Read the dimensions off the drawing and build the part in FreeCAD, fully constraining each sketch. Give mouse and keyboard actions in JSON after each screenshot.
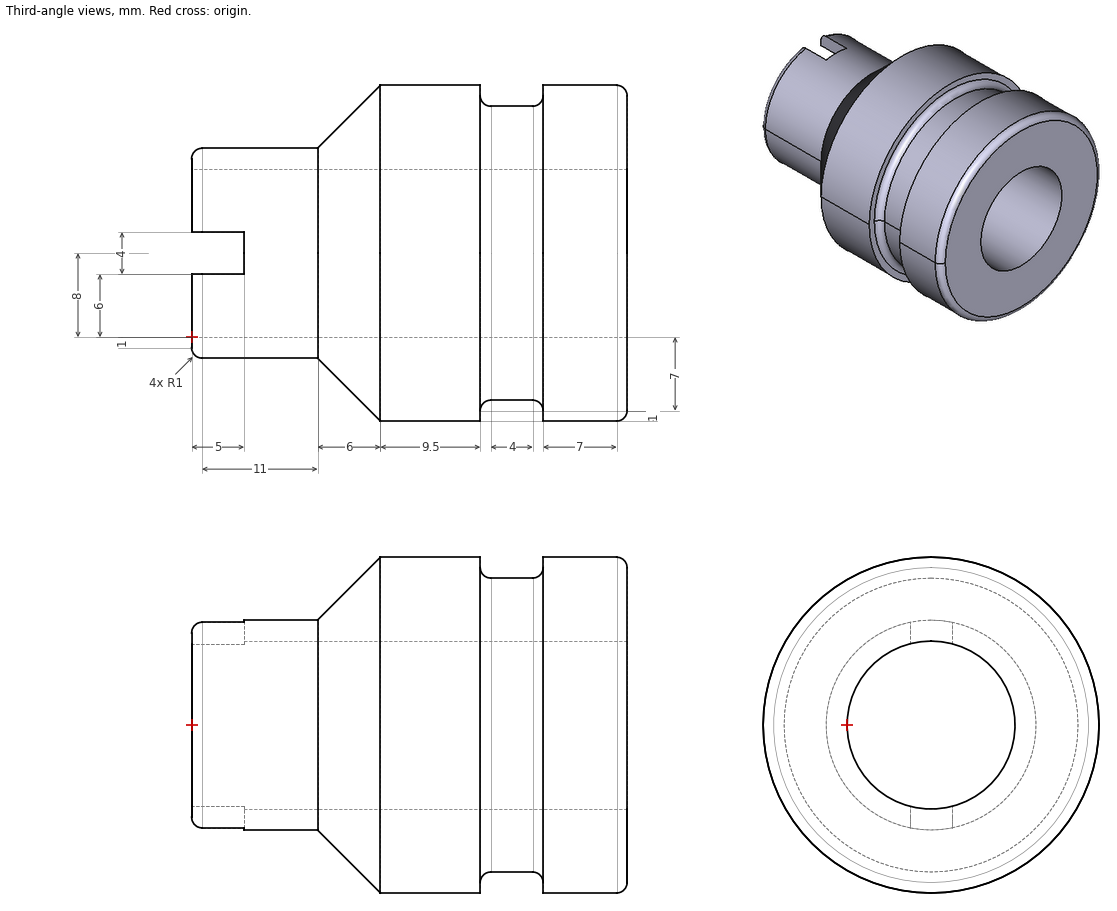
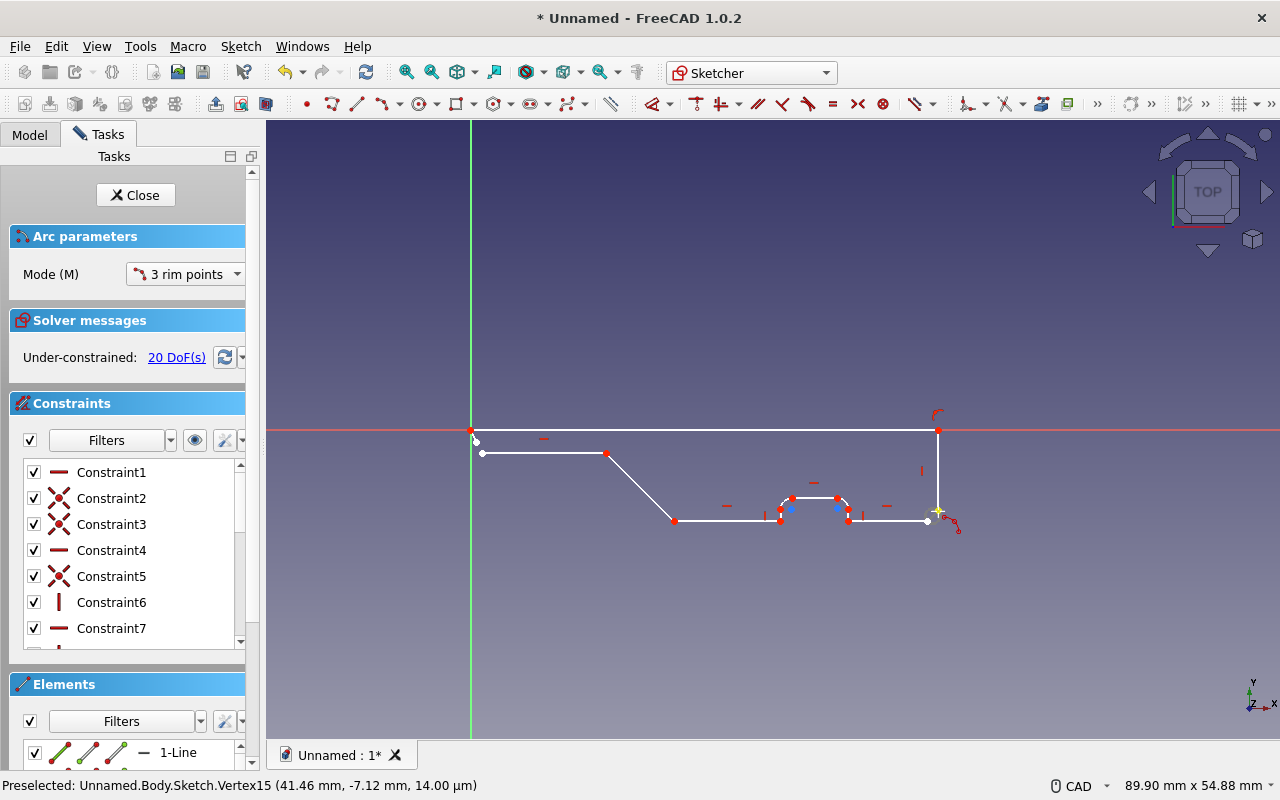
{"action": "scroll", "coordinate": [936, 517], "scroll_direction": "up", "scroll_amount": 8}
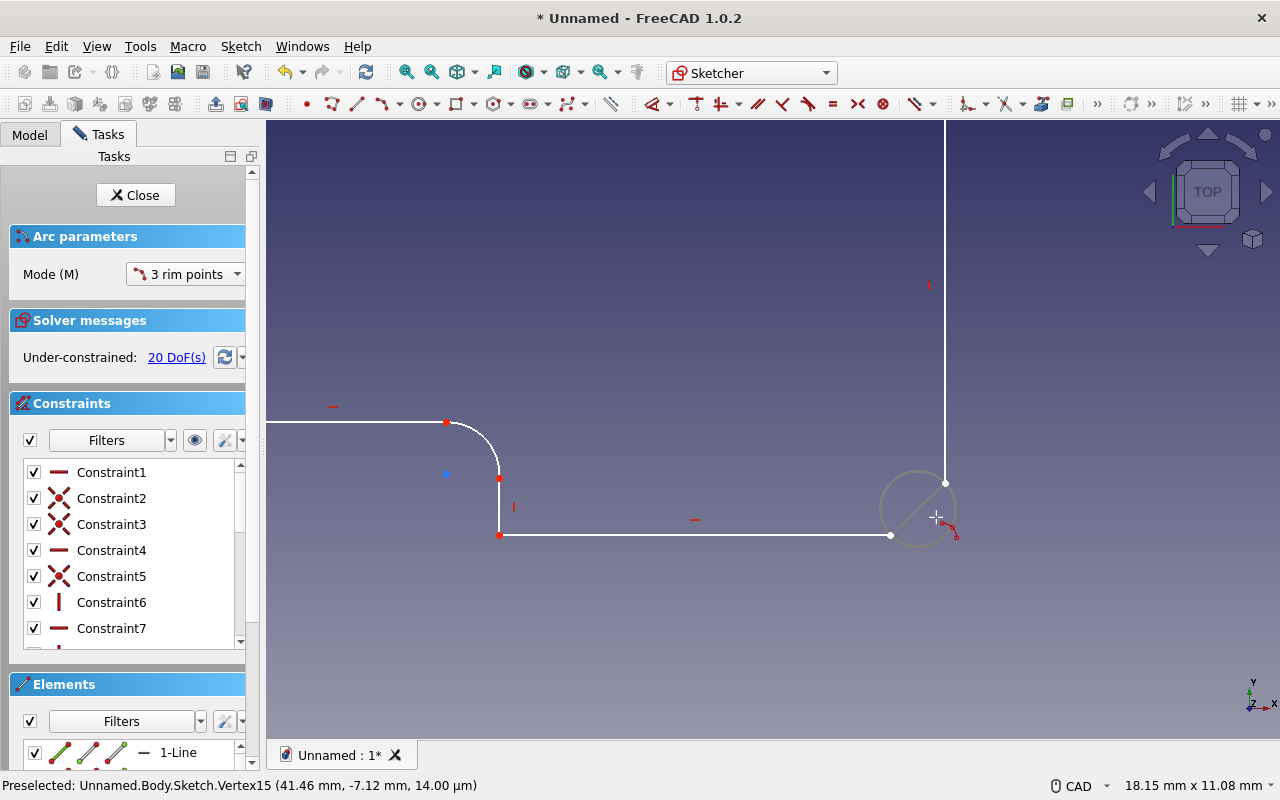
{"action": "left_click", "coordinate": [931, 516]}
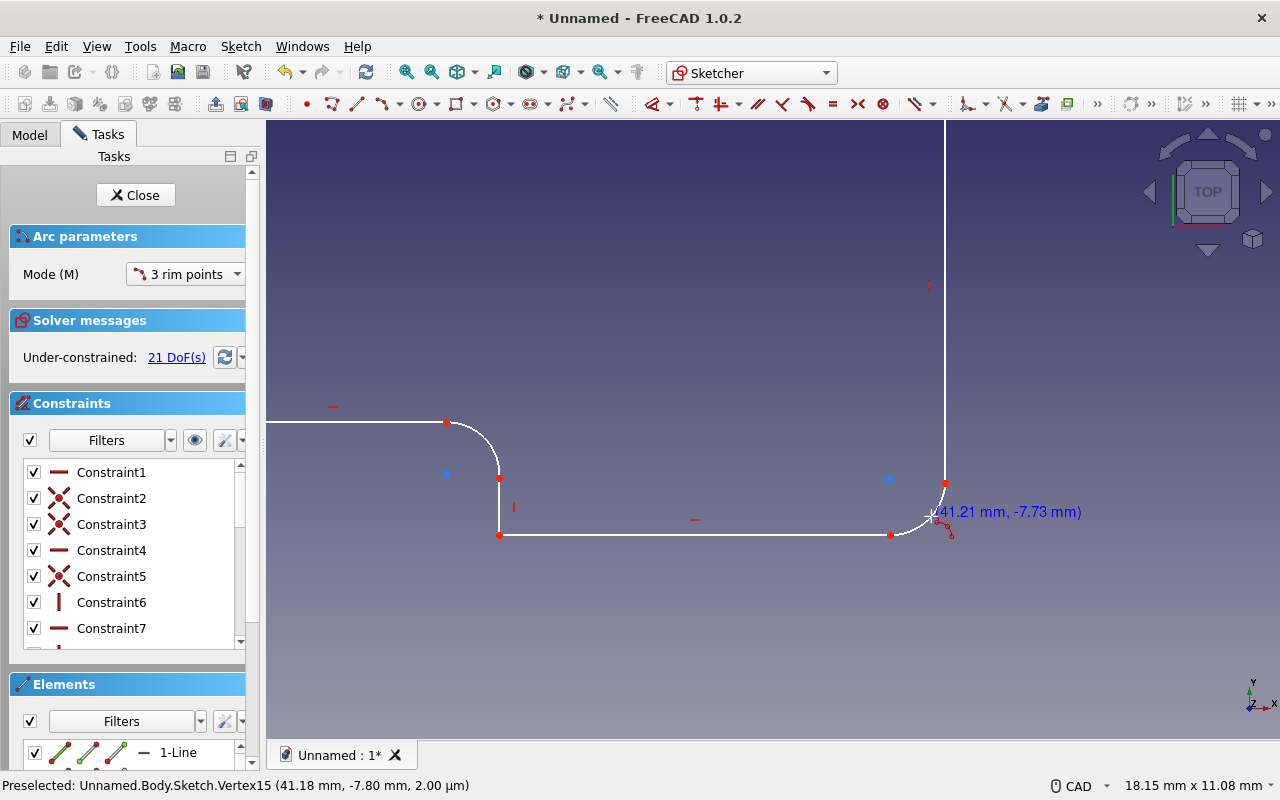
{"action": "scroll", "coordinate": [936, 517], "scroll_direction": "down", "scroll_amount": 8}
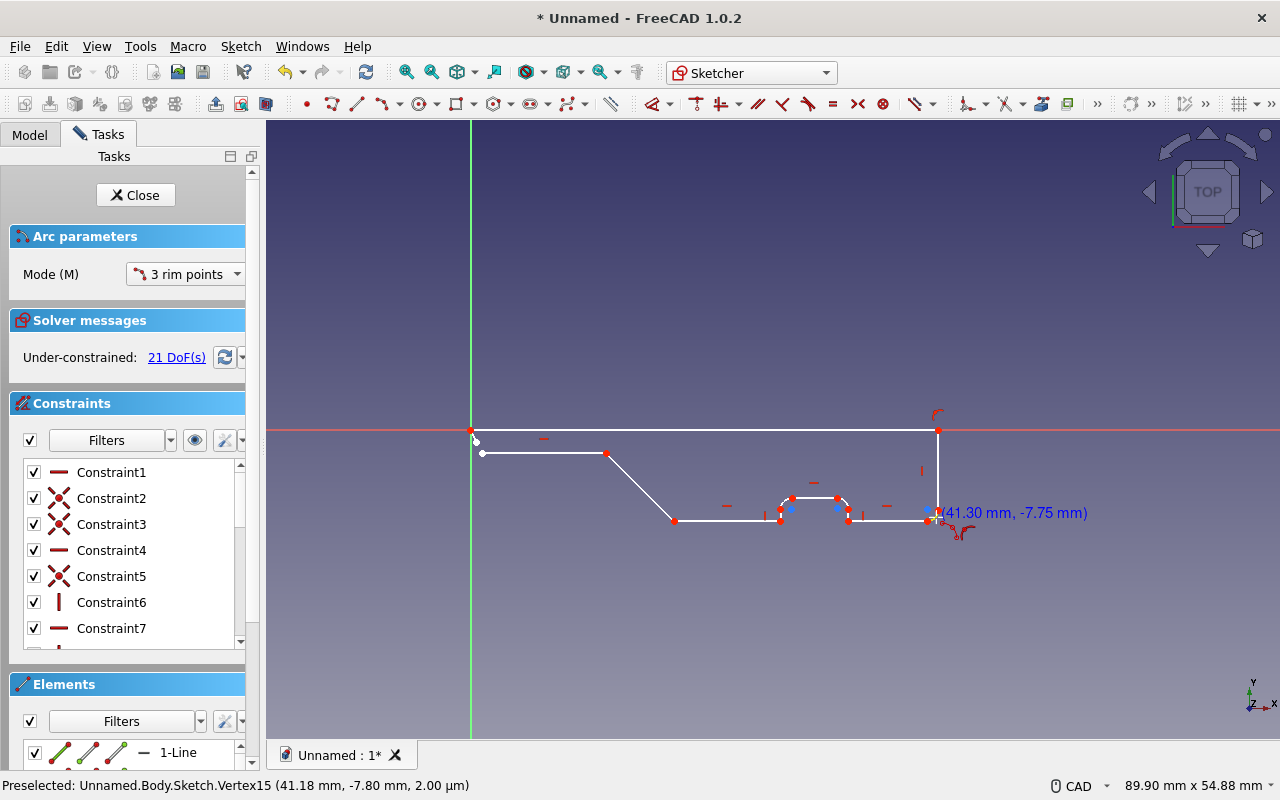
{"action": "scroll", "coordinate": [471, 442], "scroll_direction": "up", "scroll_amount": 6}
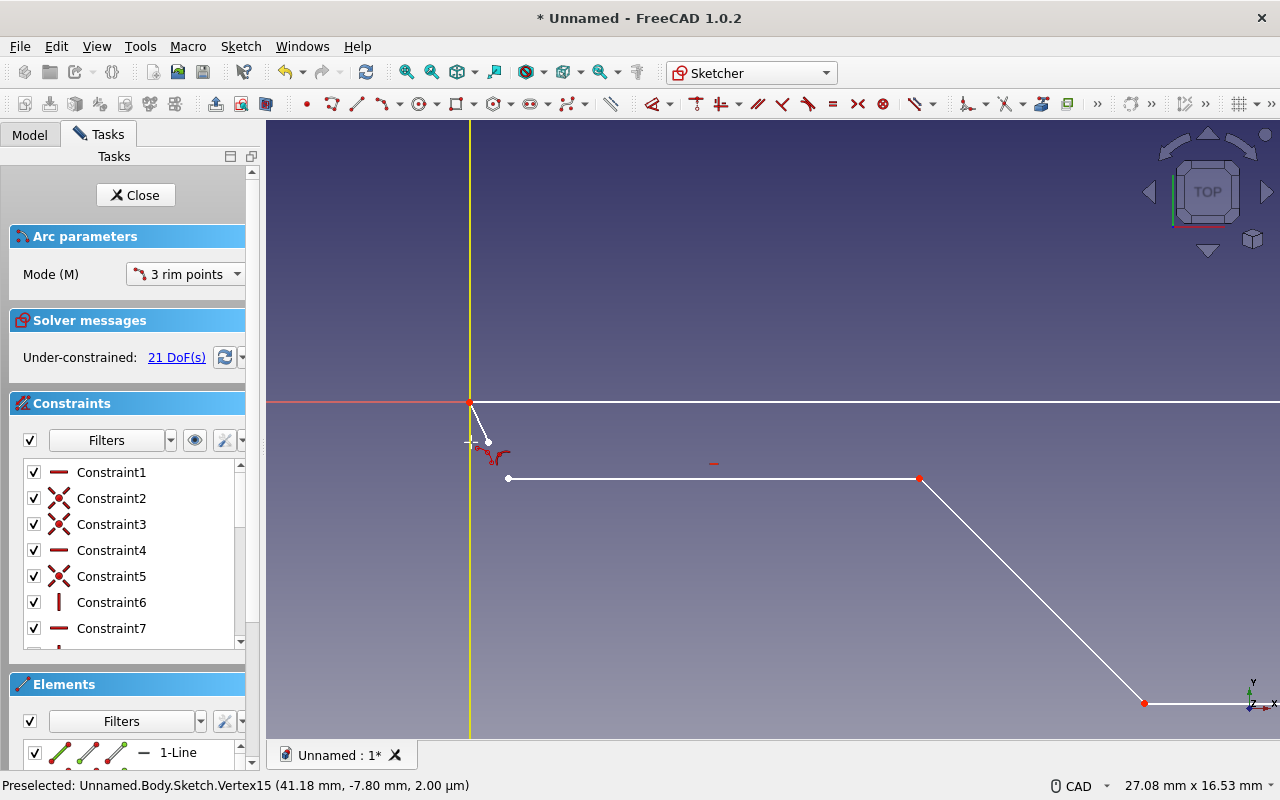
{"action": "left_click", "coordinate": [489, 442]}
{"action": "left_click", "coordinate": [508, 479]}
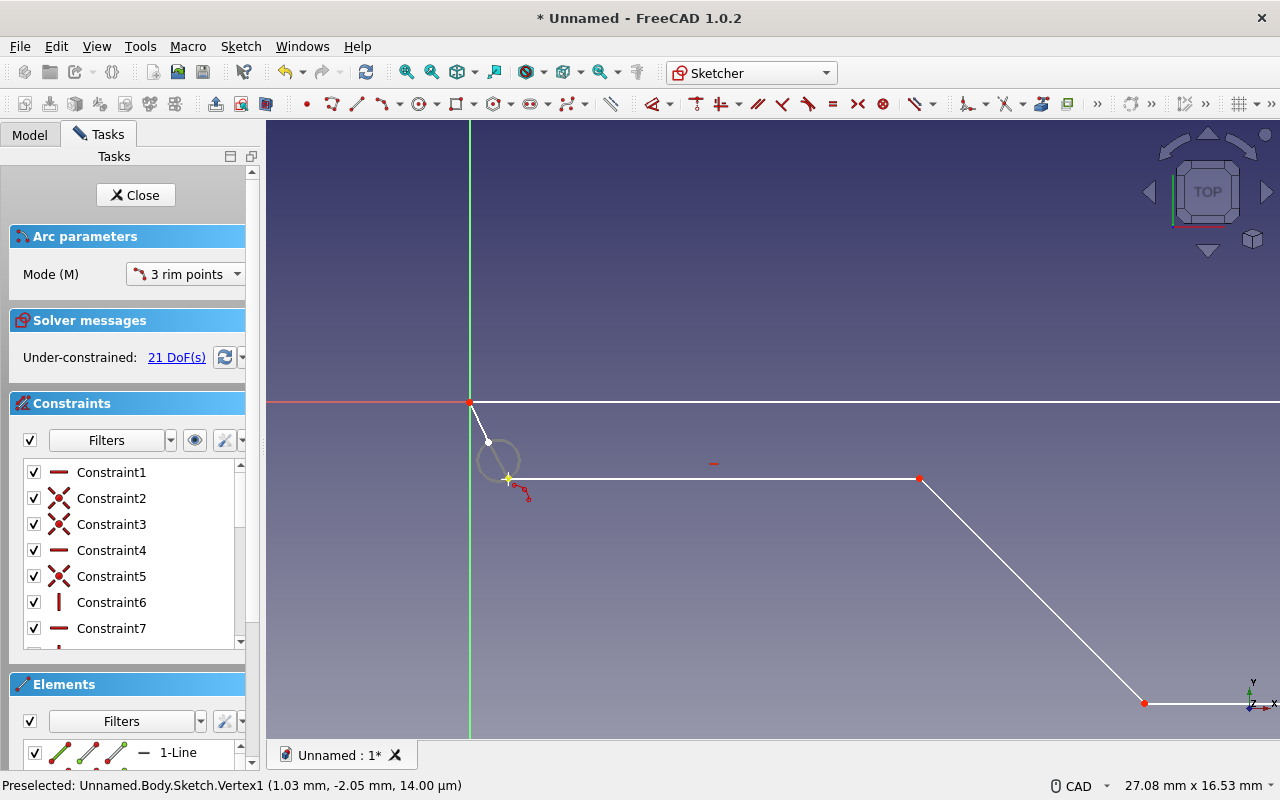
{"action": "scroll", "coordinate": [481, 466], "scroll_direction": "up", "scroll_amount": 2}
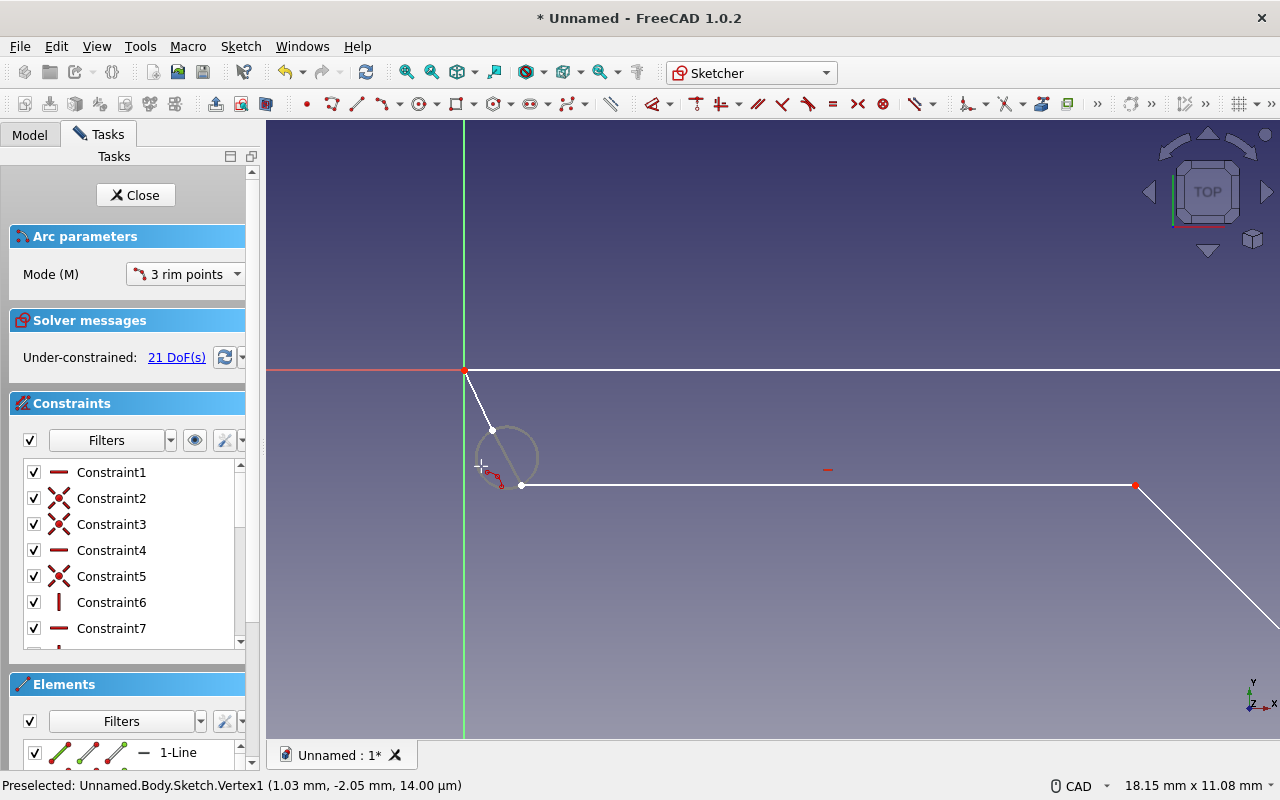
{"action": "left_click", "coordinate": [480, 466]}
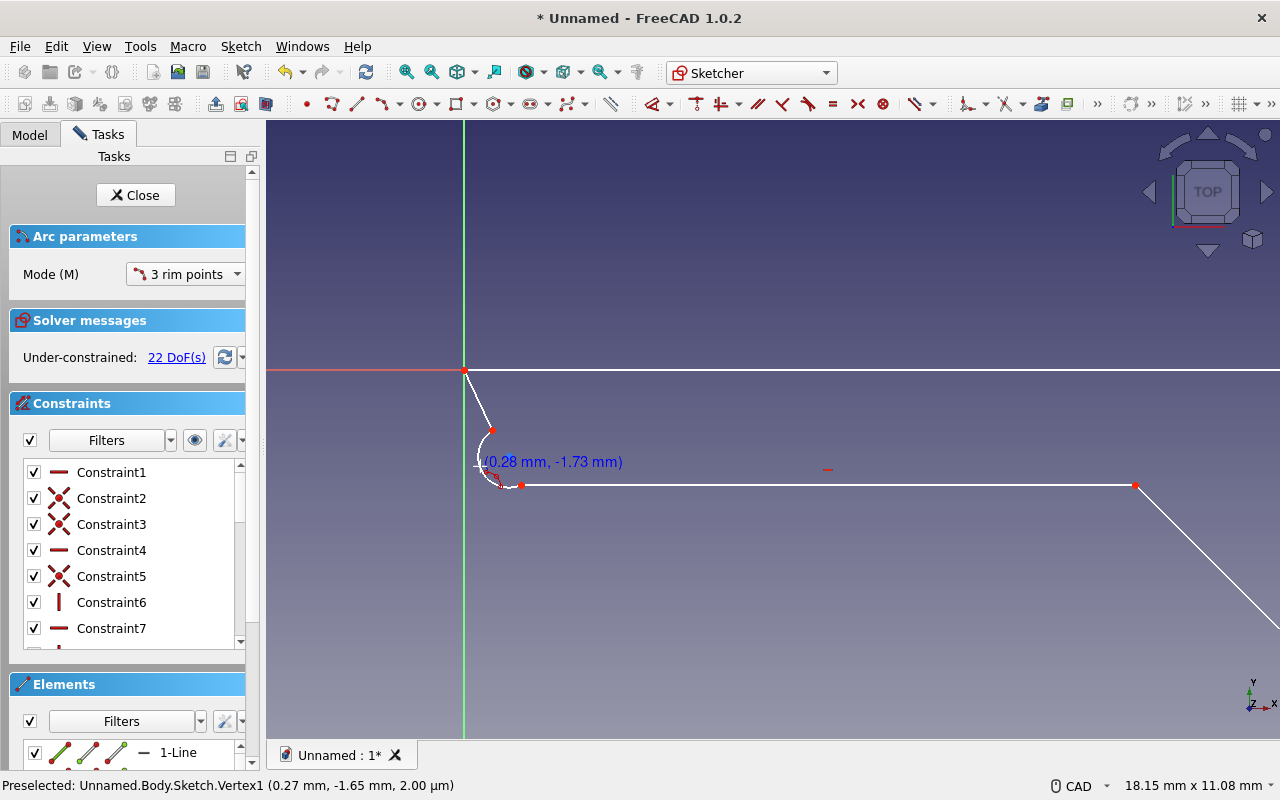
{"action": "key", "text": "g l"}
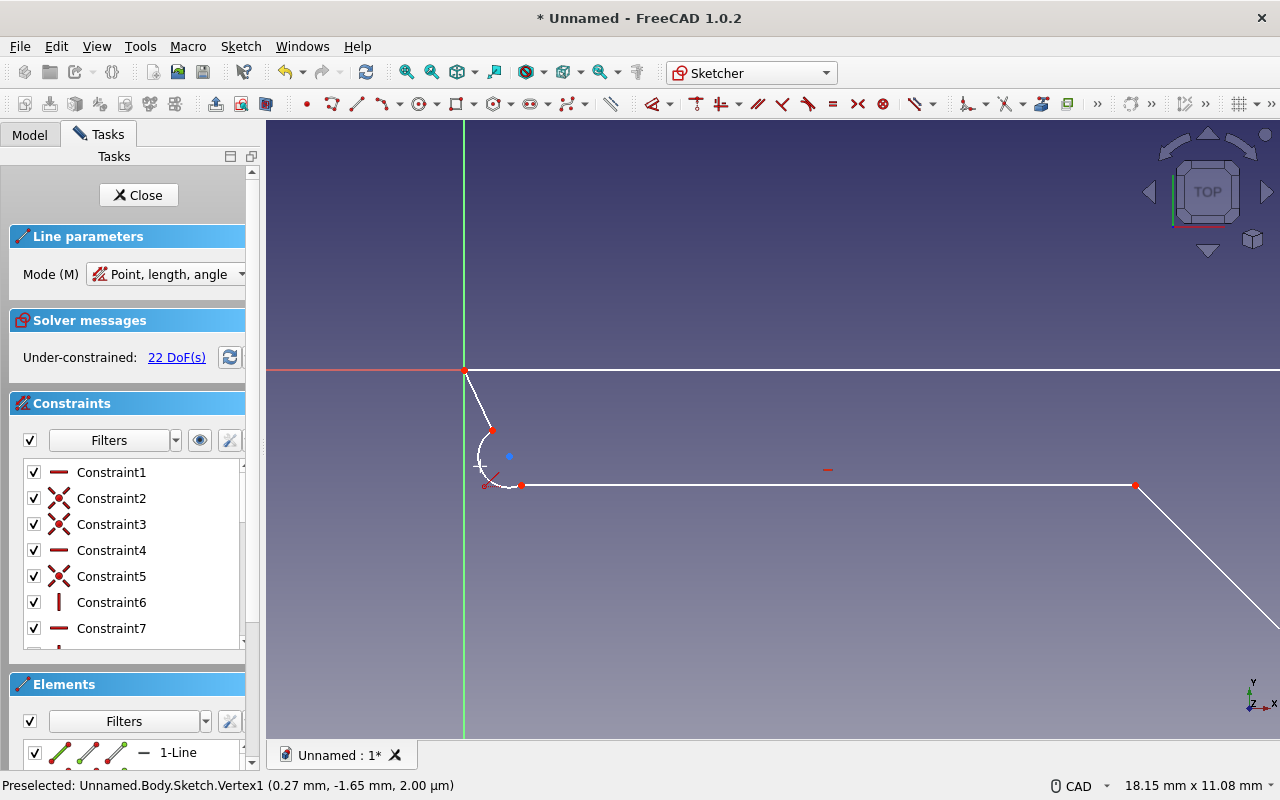
{"action": "scroll", "coordinate": [472, 444], "scroll_direction": "down", "scroll_amount": 8}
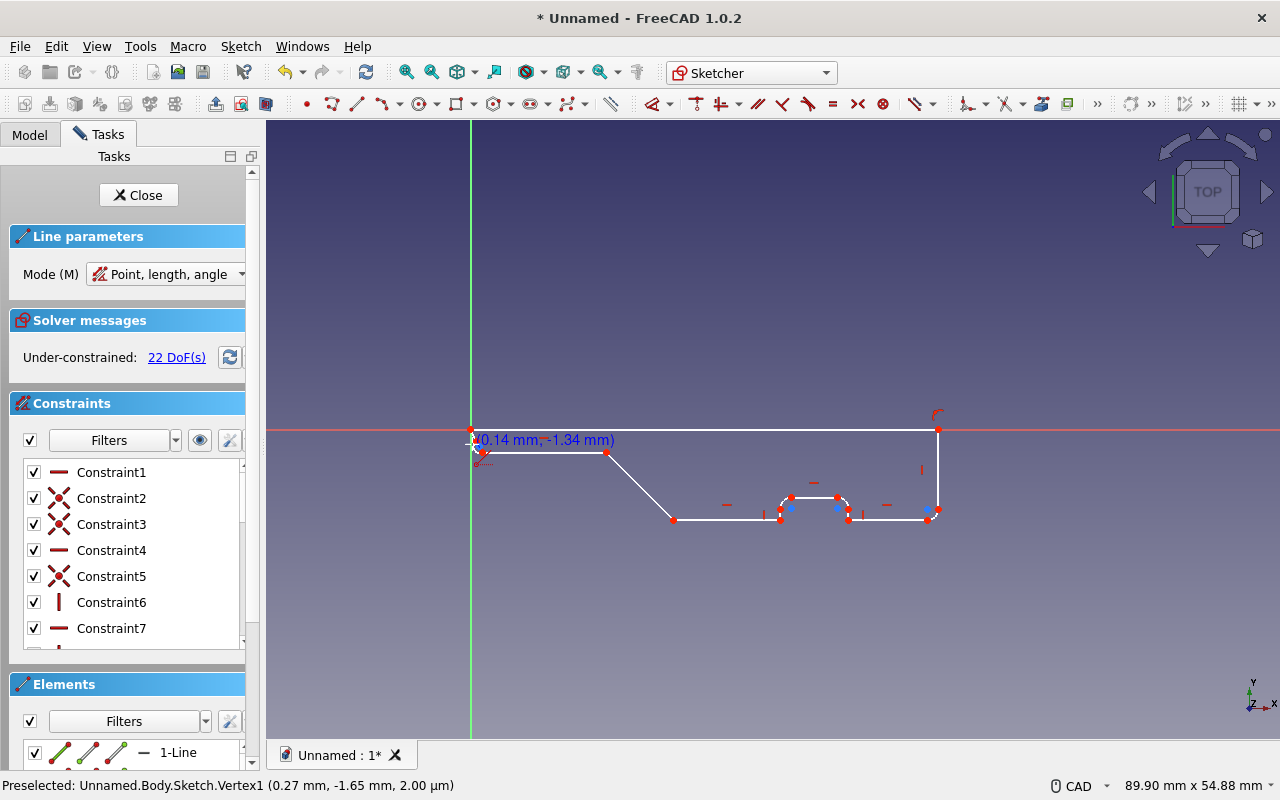
{"action": "left_click", "coordinate": [424, 339]}
{"action": "left_click", "coordinate": [985, 339]}
{"action": "key", "text": "Escape"}